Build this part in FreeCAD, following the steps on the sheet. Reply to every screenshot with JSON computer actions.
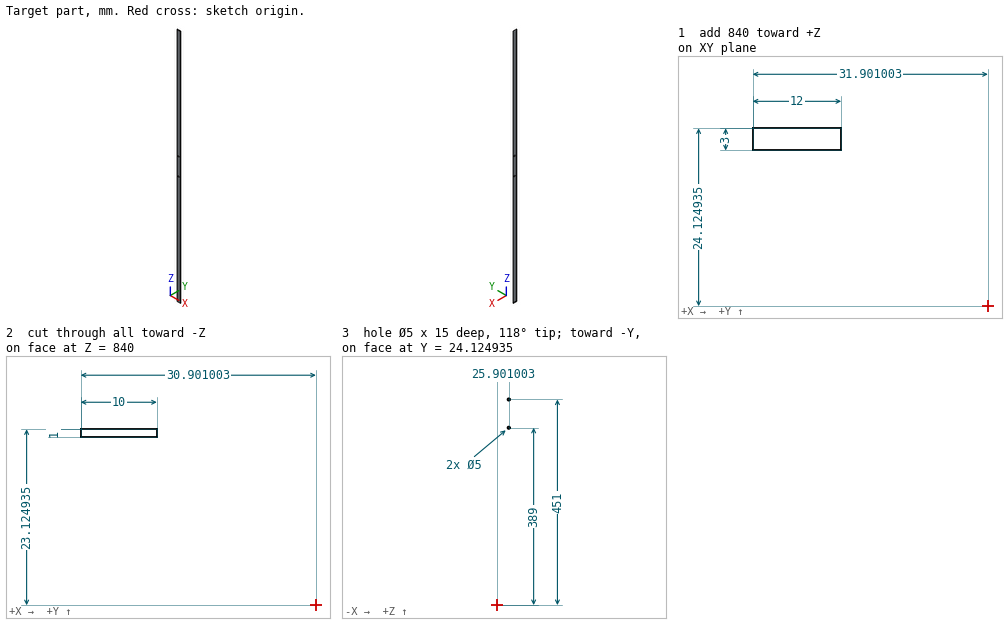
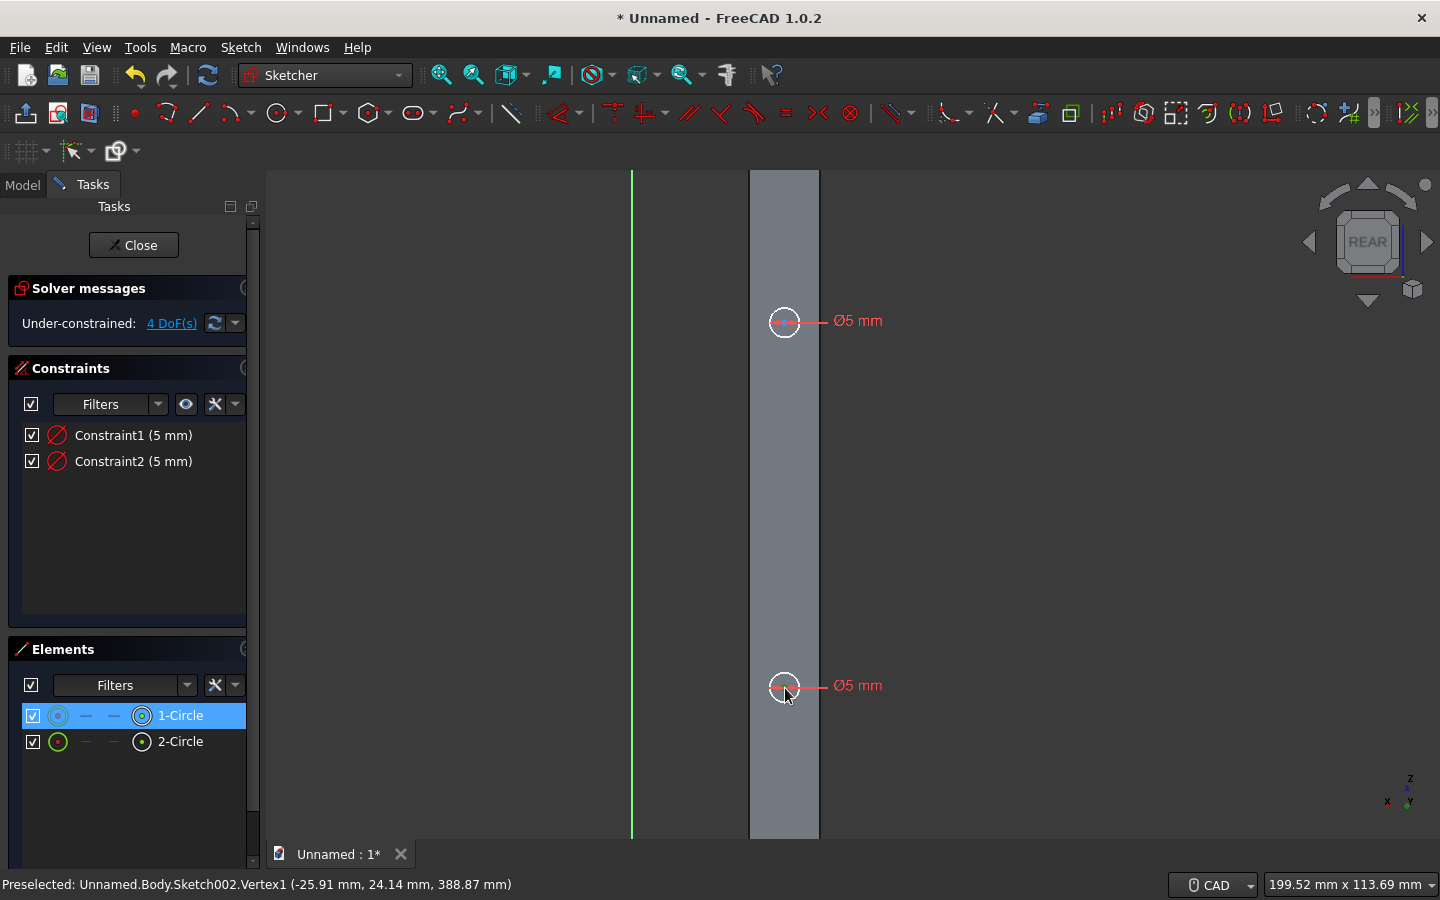
{"action": "left_click", "coordinate": [785, 323]}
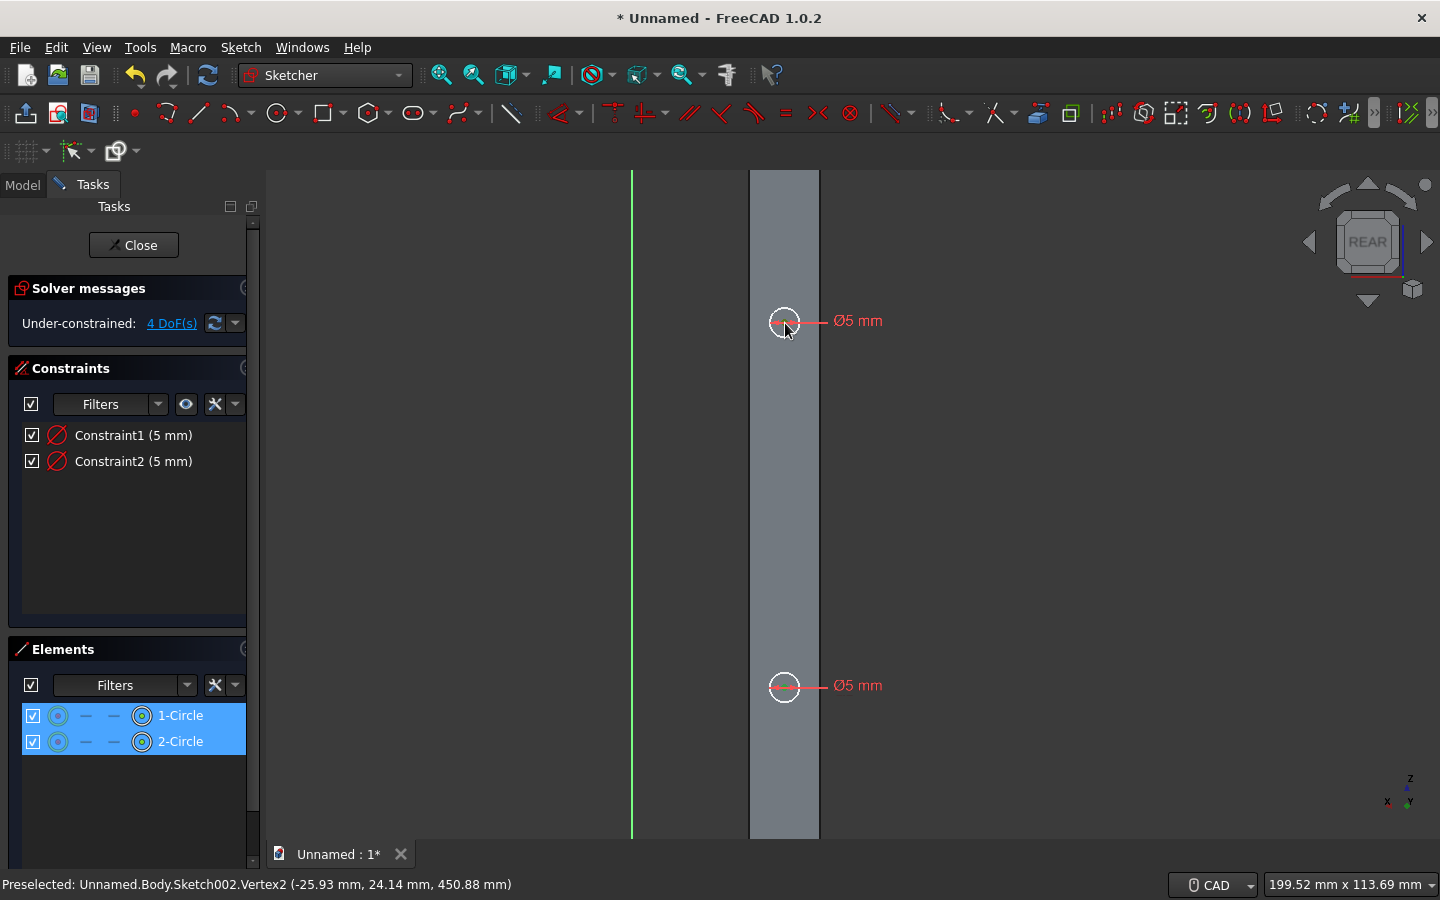
{"action": "key", "text": "v"}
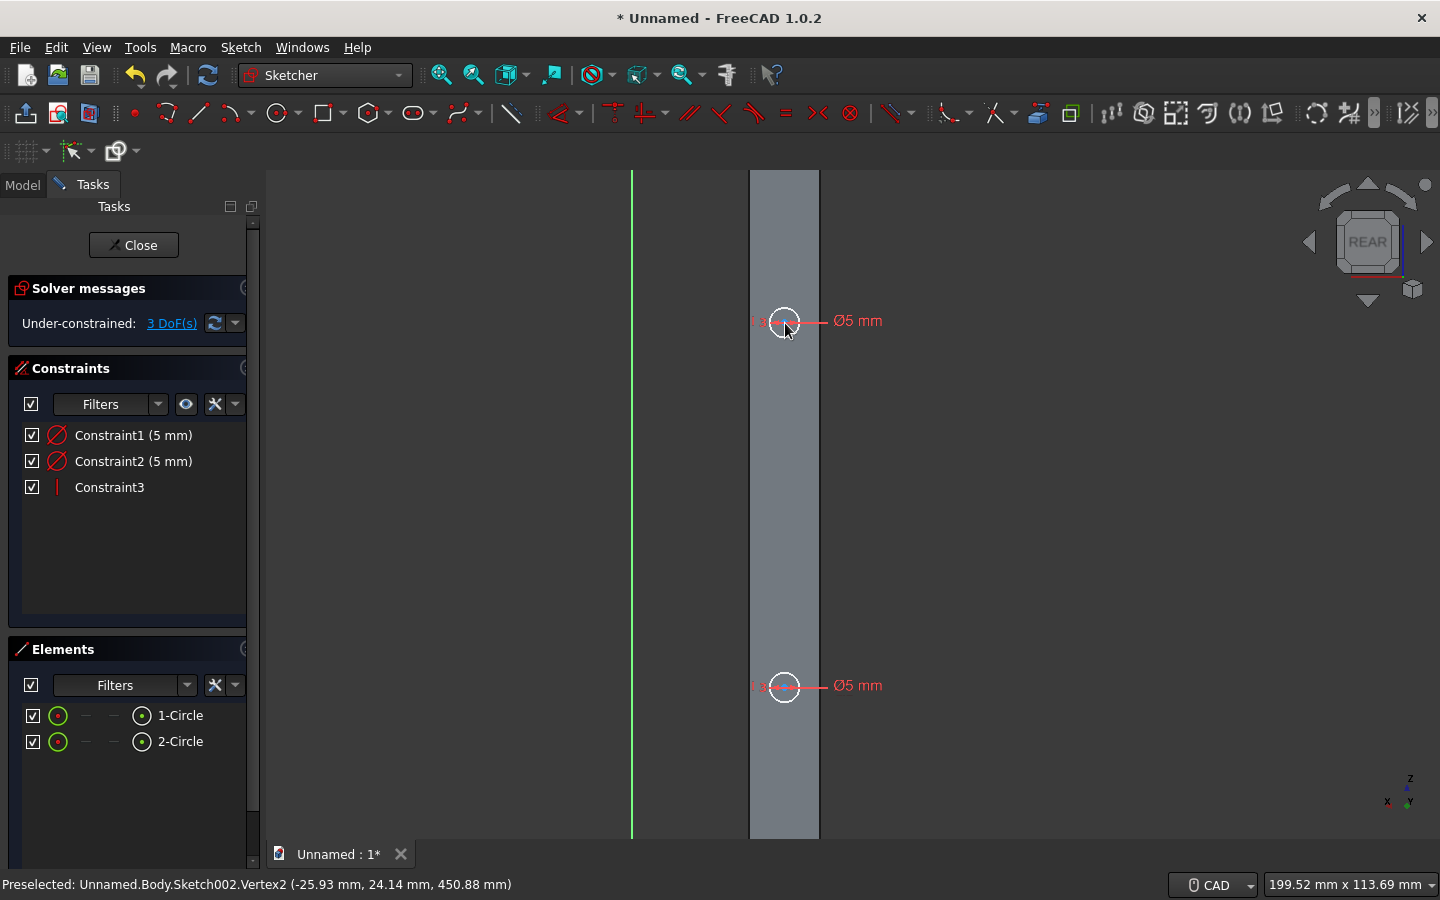
{"action": "left_click", "coordinate": [558, 114]}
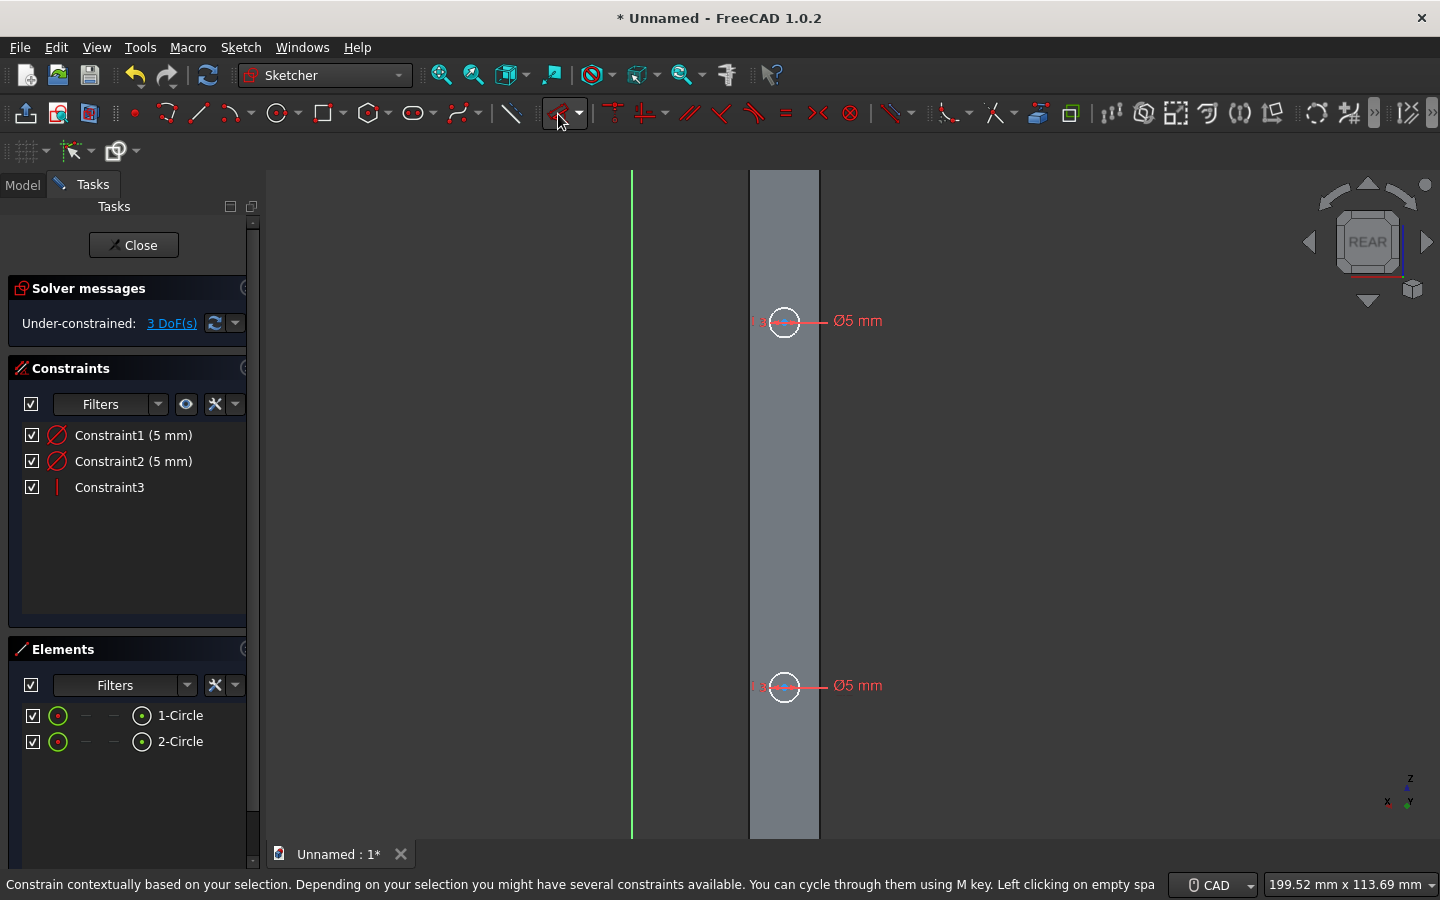
{"action": "left_click", "coordinate": [785, 688]}
{"action": "left_click", "coordinate": [598, 749]}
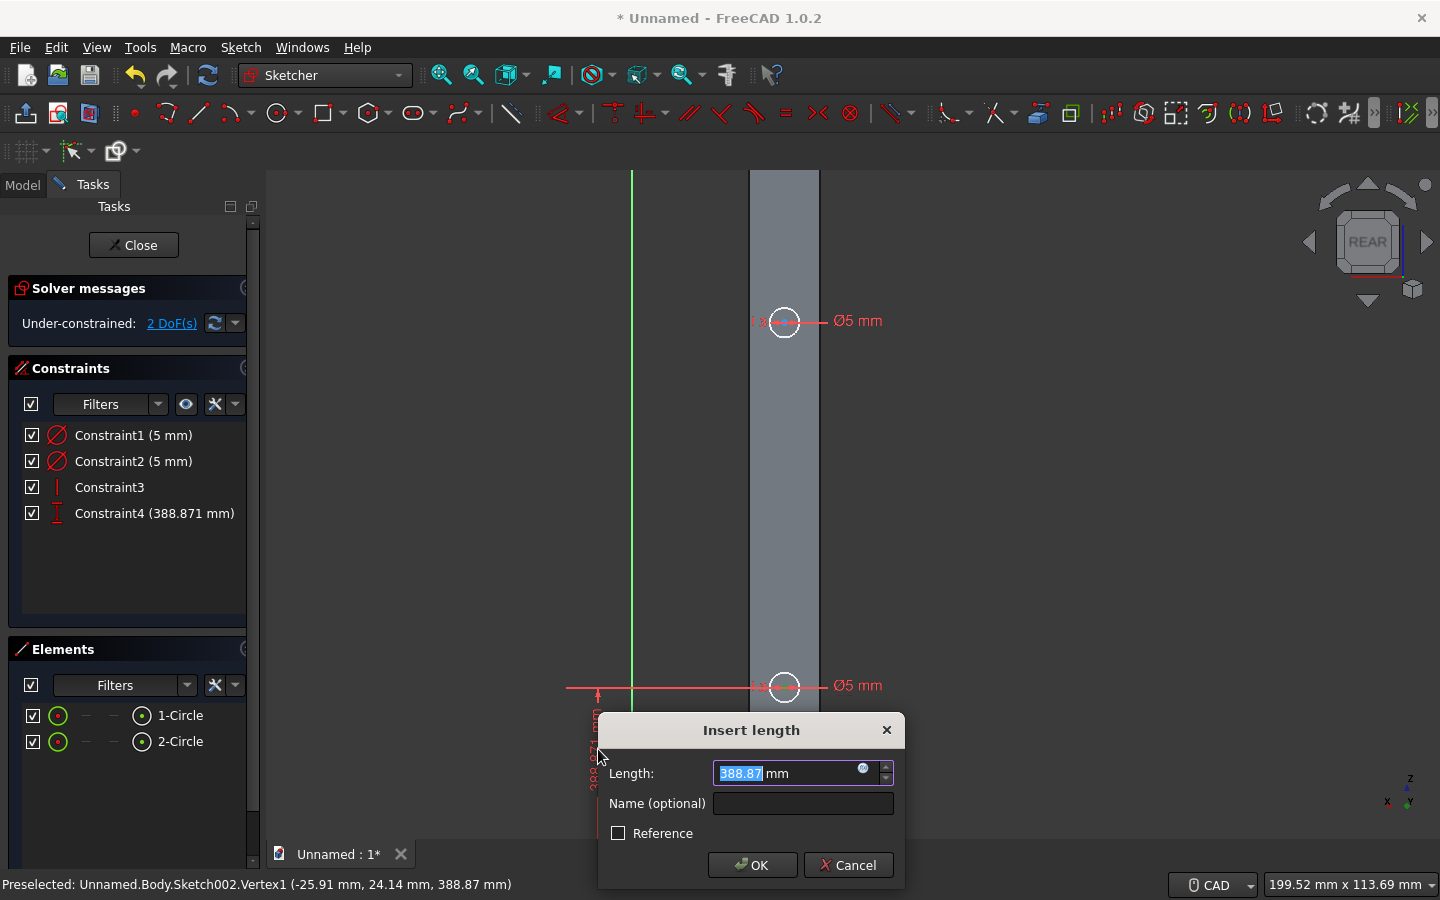
{"action": "type", "text": "389"}
{"action": "key", "text": "Return"}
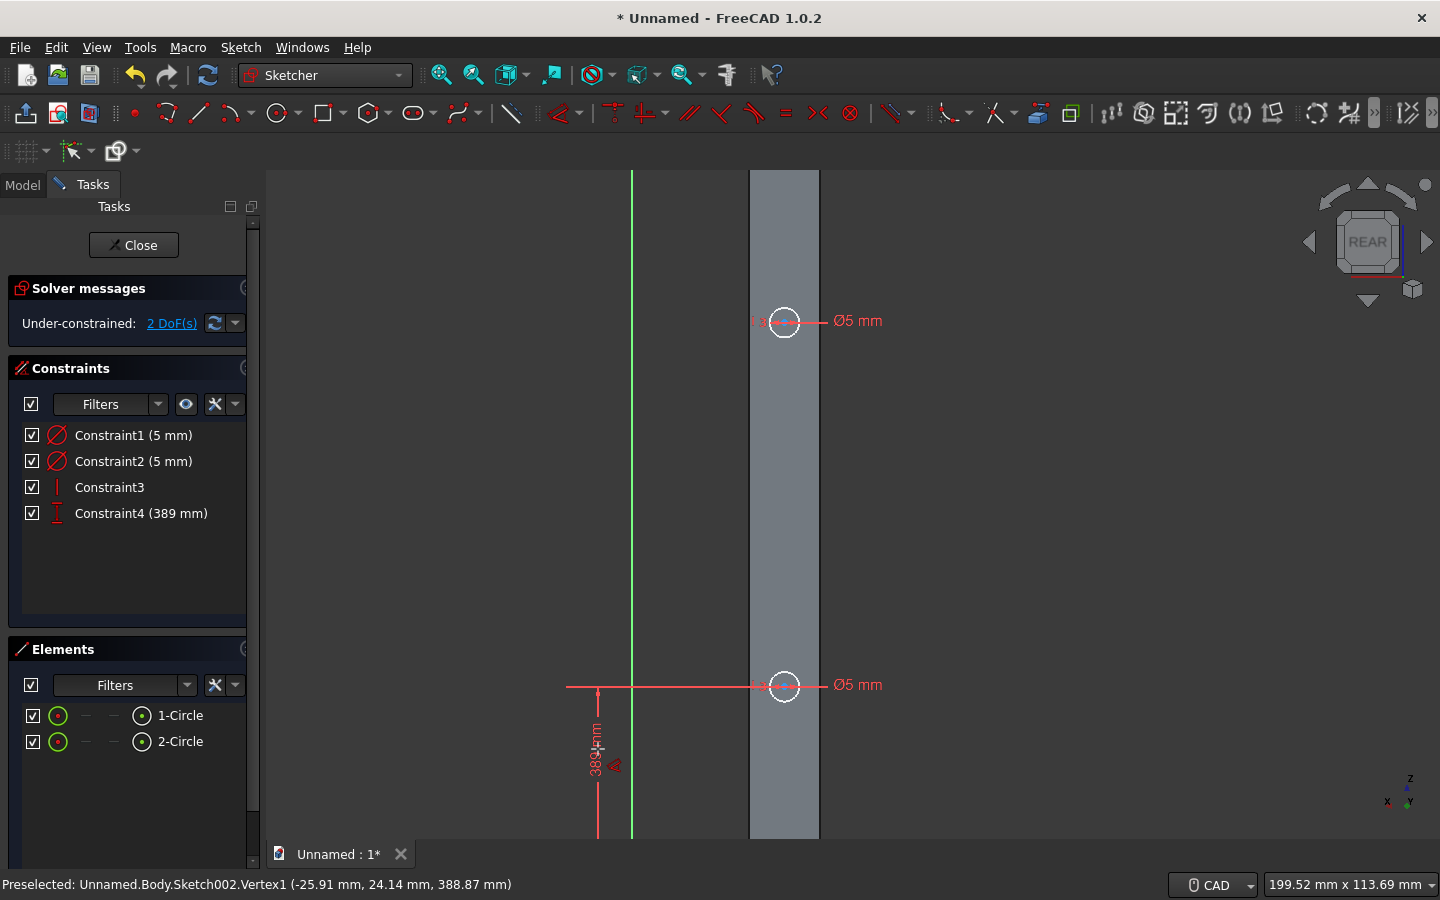
{"action": "left_click", "coordinate": [785, 323]}
{"action": "left_click", "coordinate": [598, 567]}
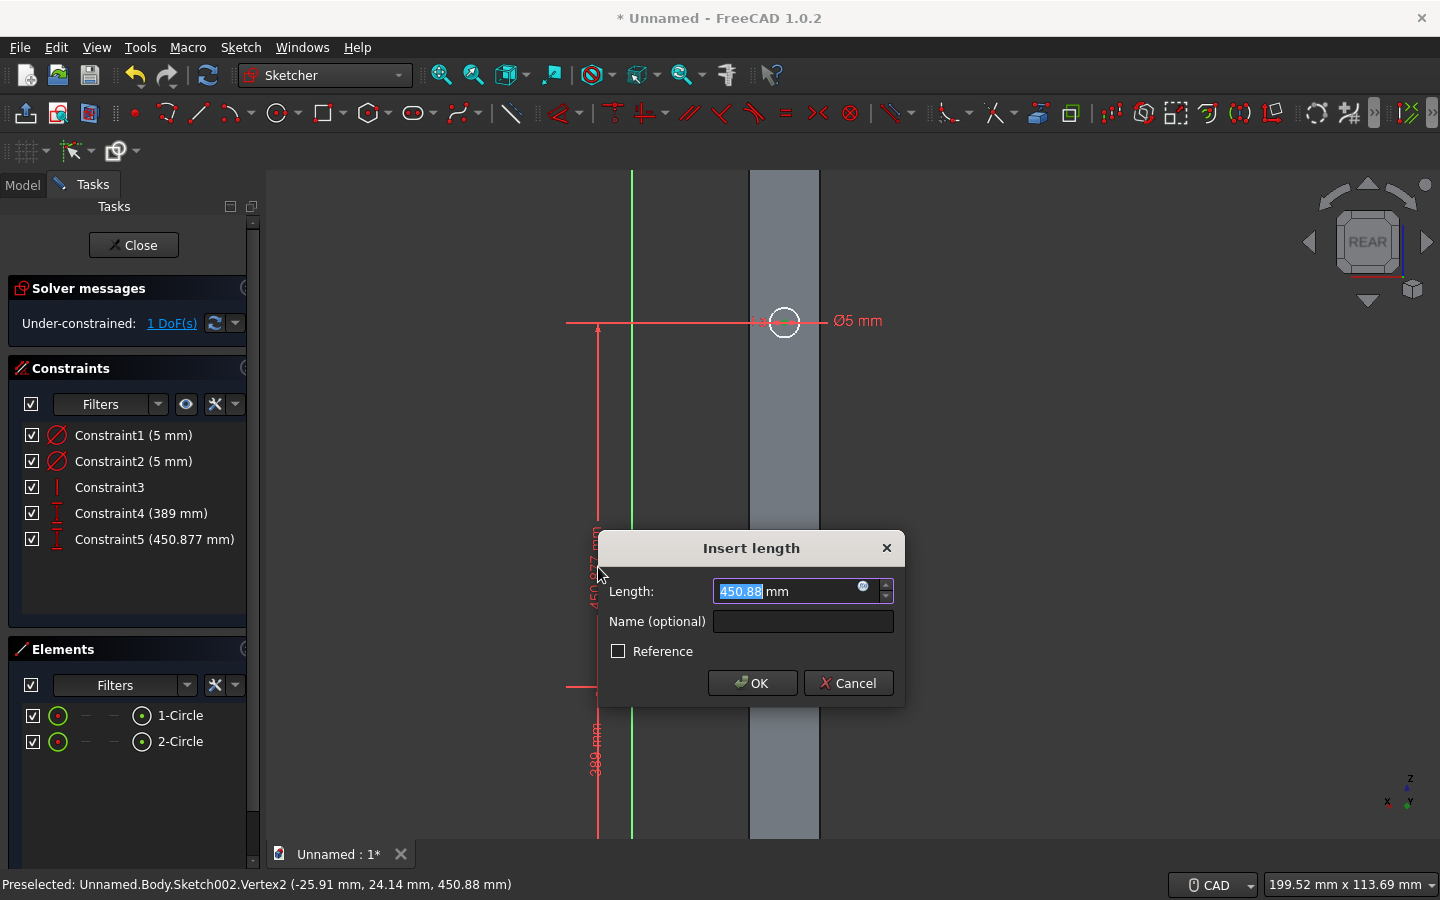
{"action": "type", "text": "451"}
{"action": "key", "text": "Return"}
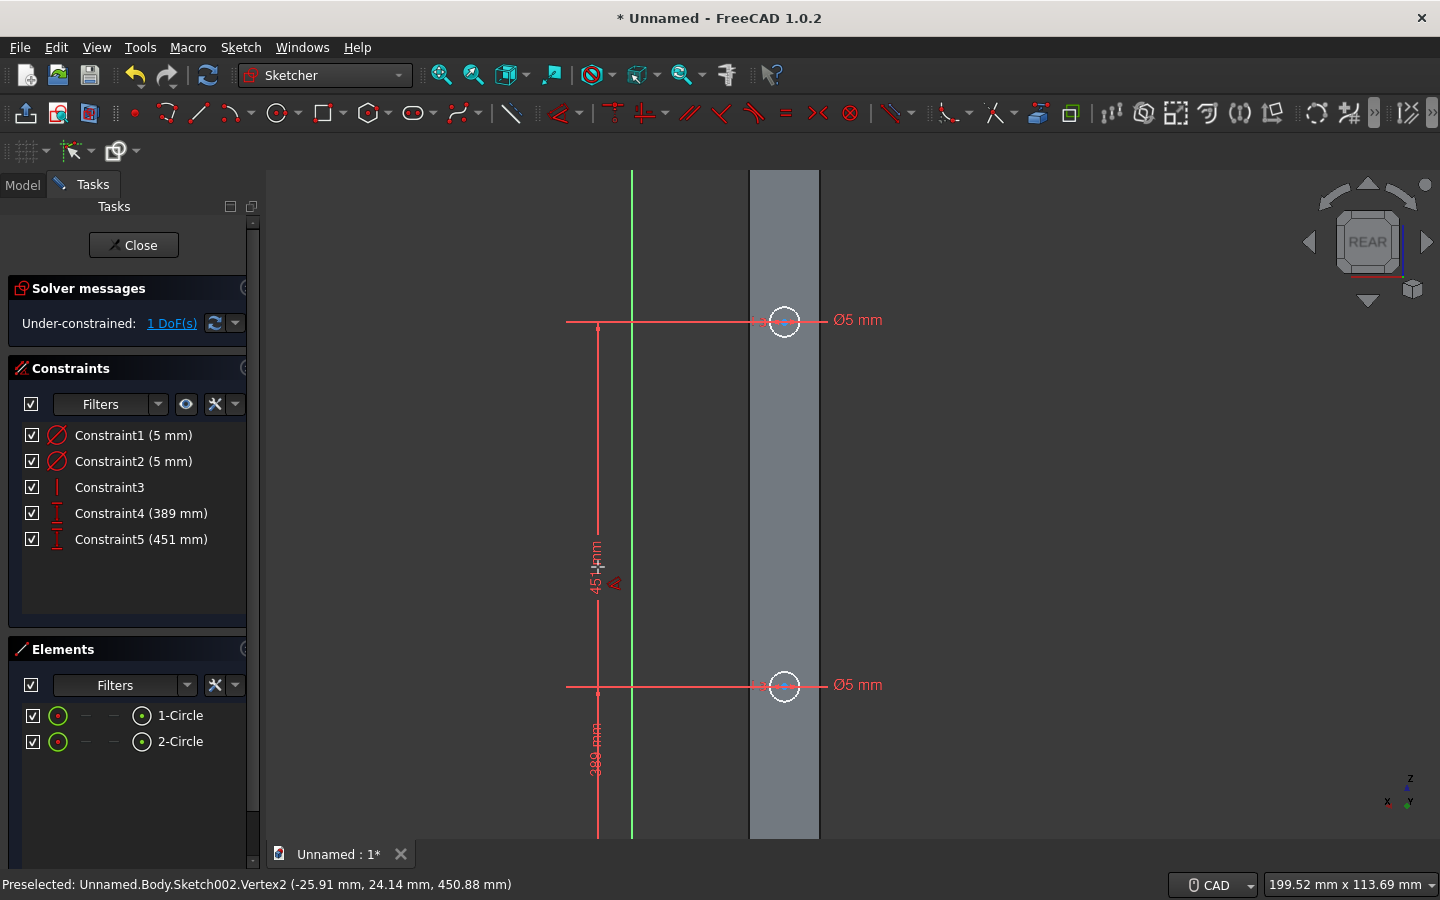
{"action": "left_click", "coordinate": [785, 687]}
{"action": "left_click", "coordinate": [708, 653]}